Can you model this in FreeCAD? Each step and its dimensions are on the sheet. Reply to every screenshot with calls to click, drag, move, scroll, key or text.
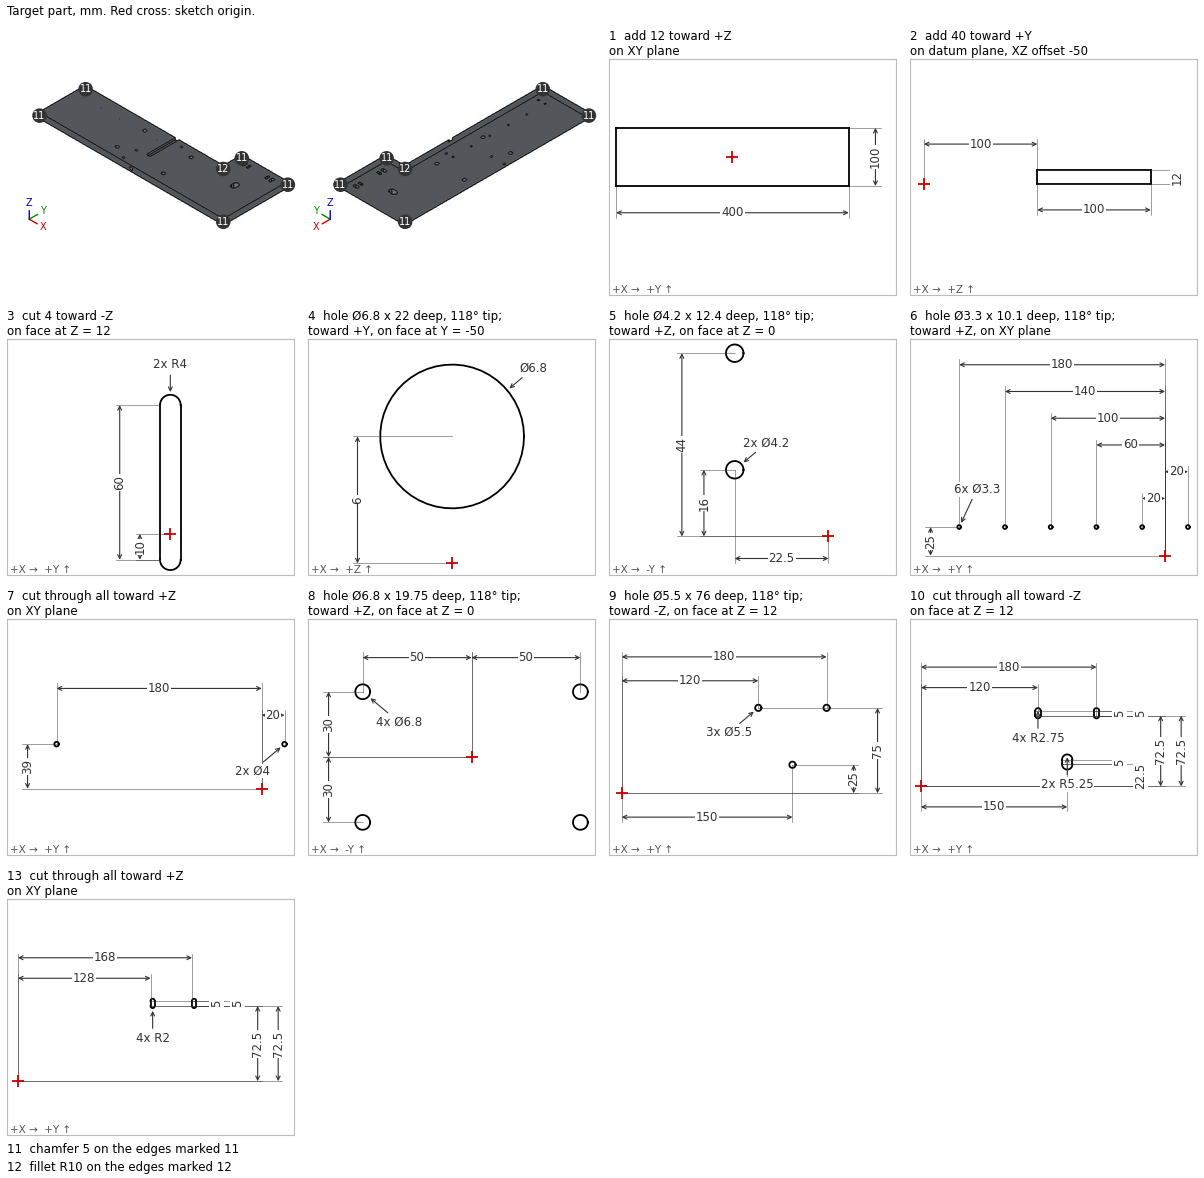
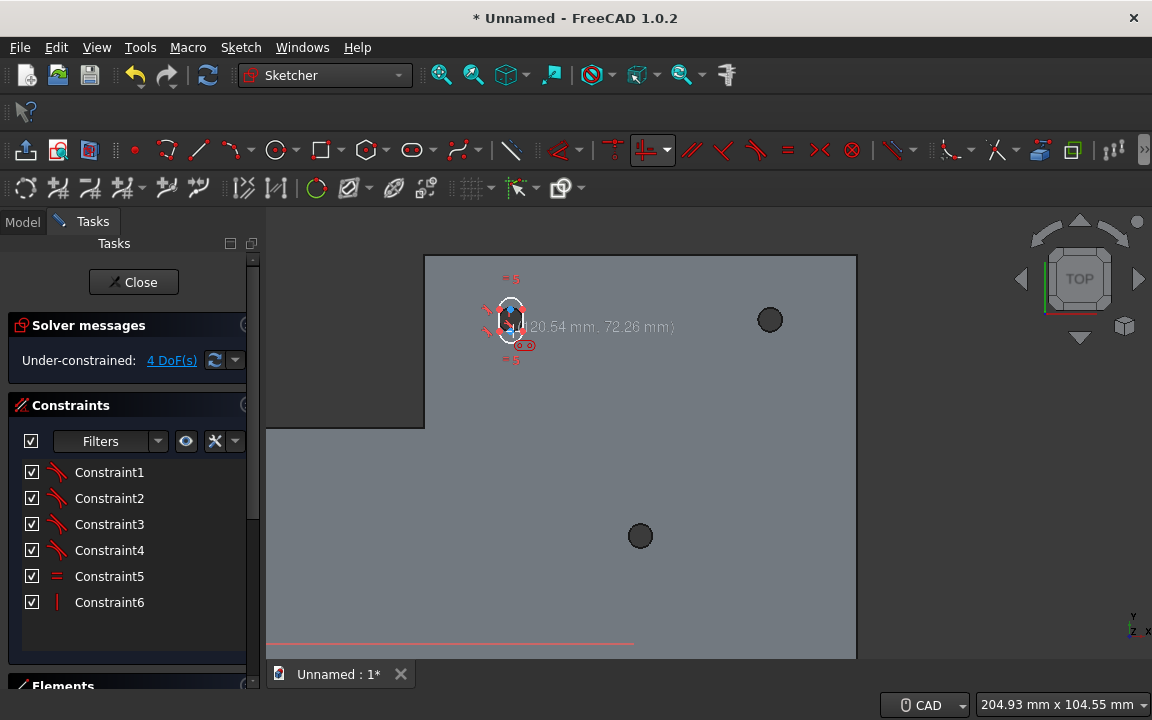
scroll(770, 331, up, 4)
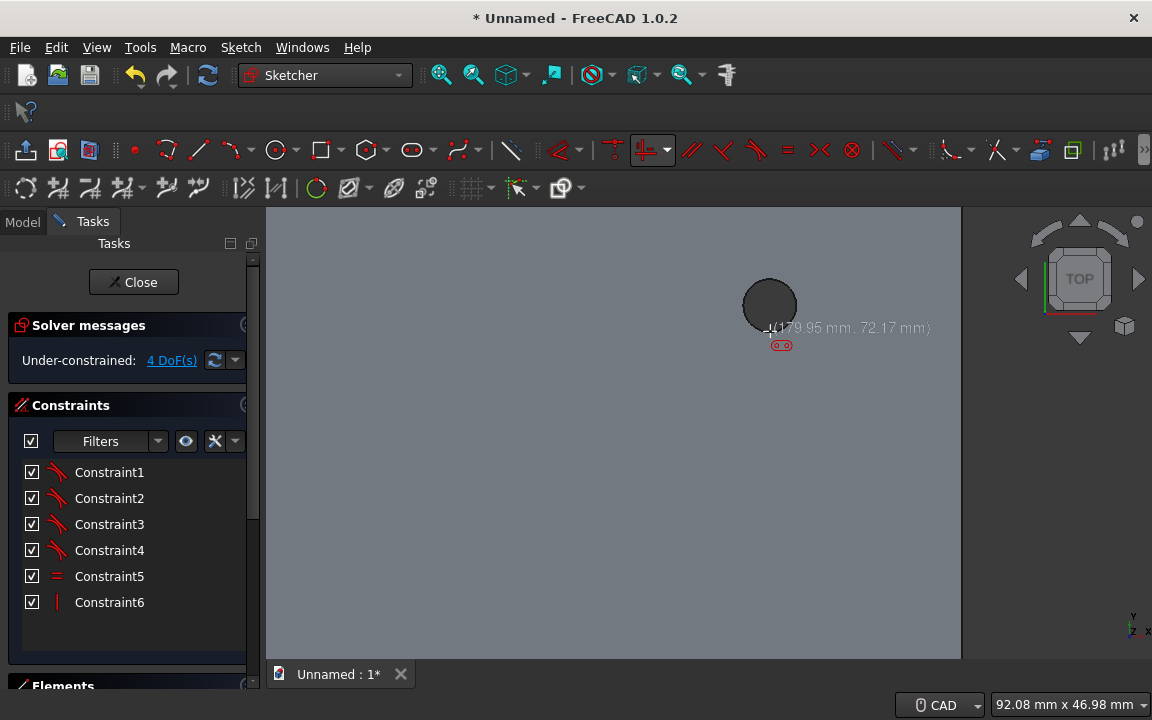
click(770, 330)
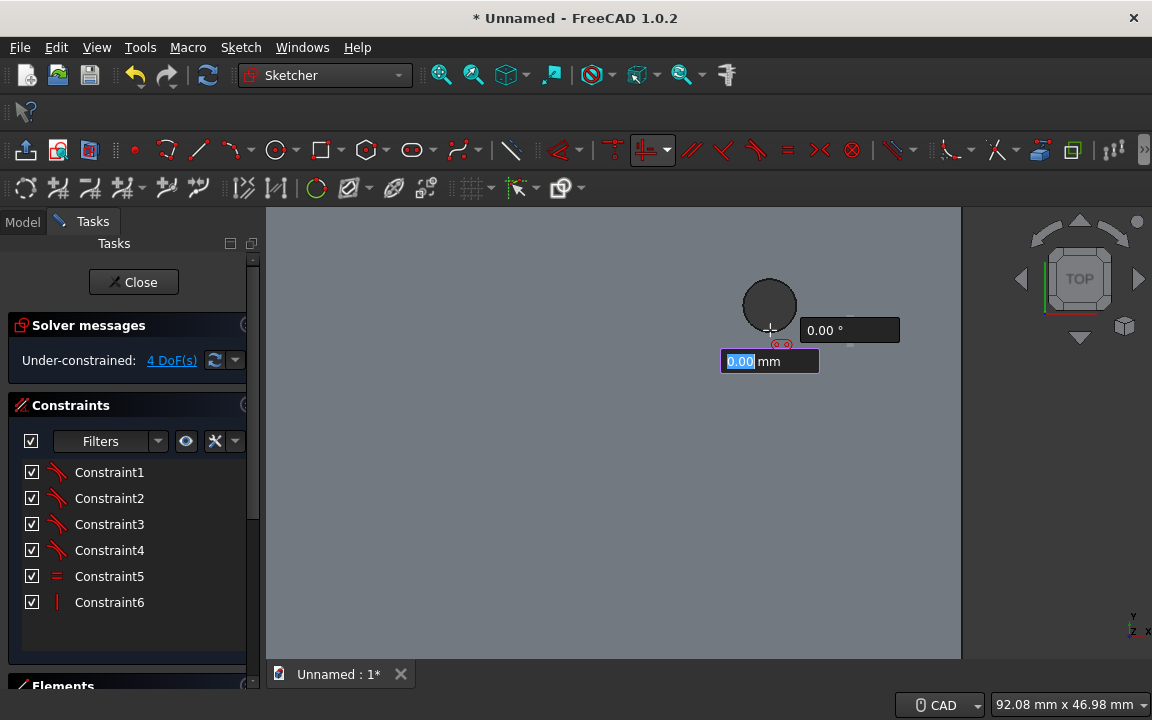
click(770, 282)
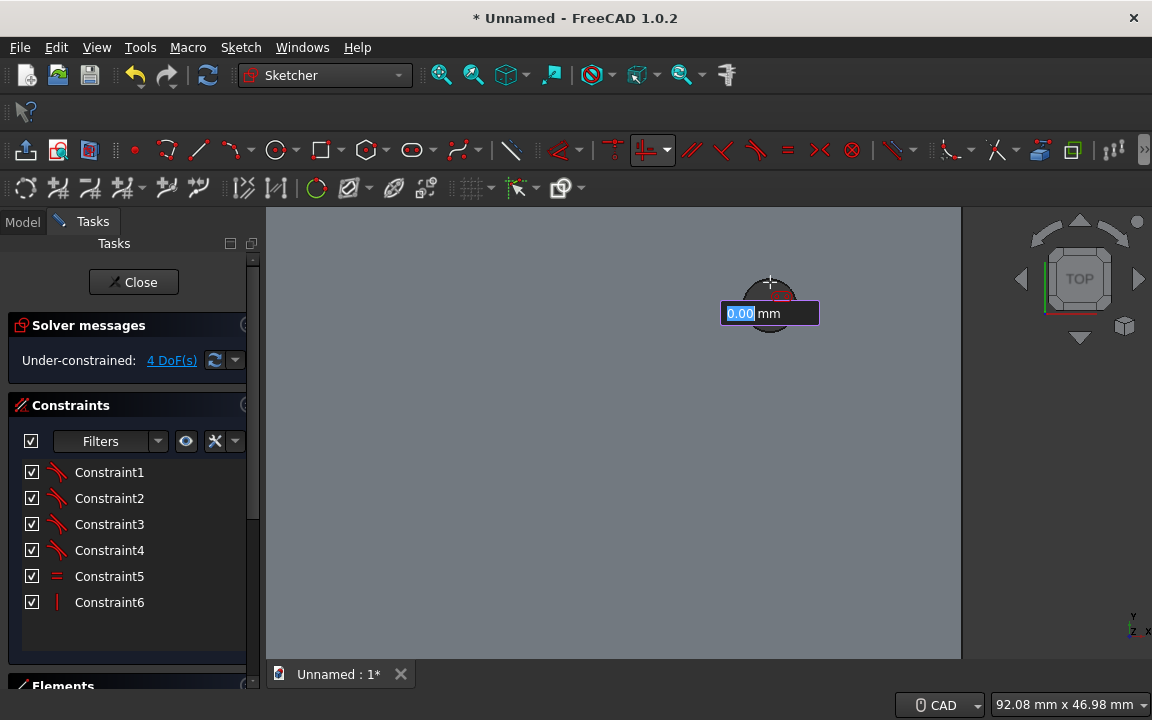
click(796, 306)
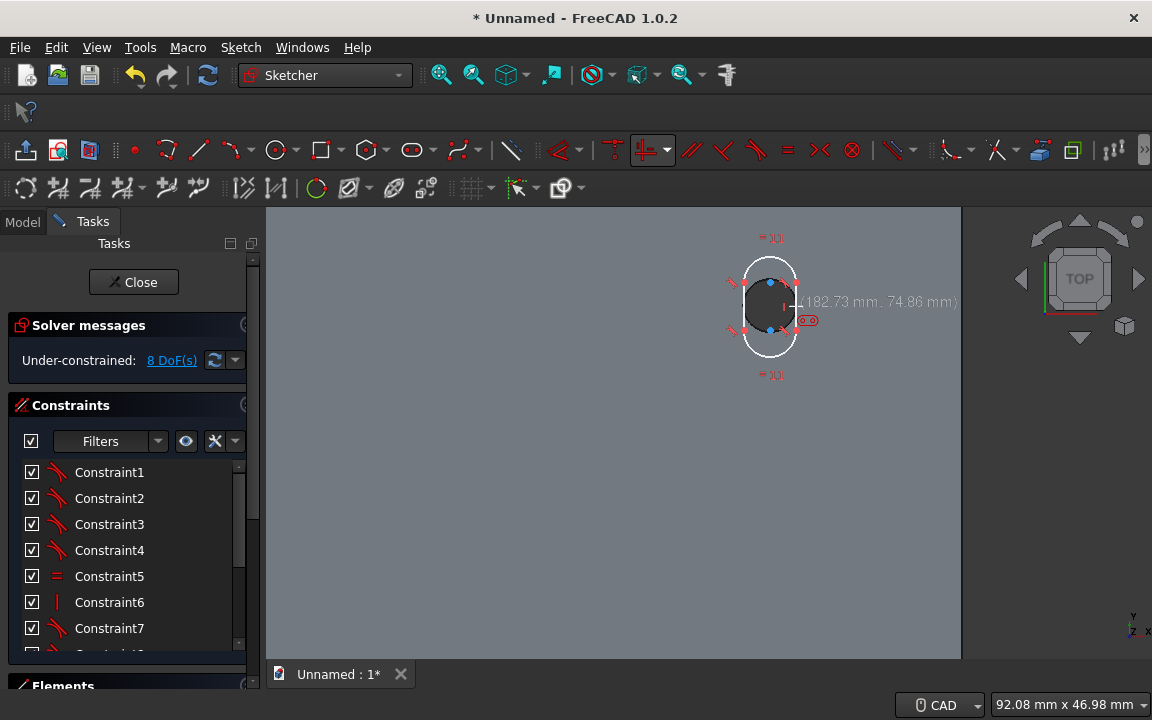
scroll(771, 331, down, 4)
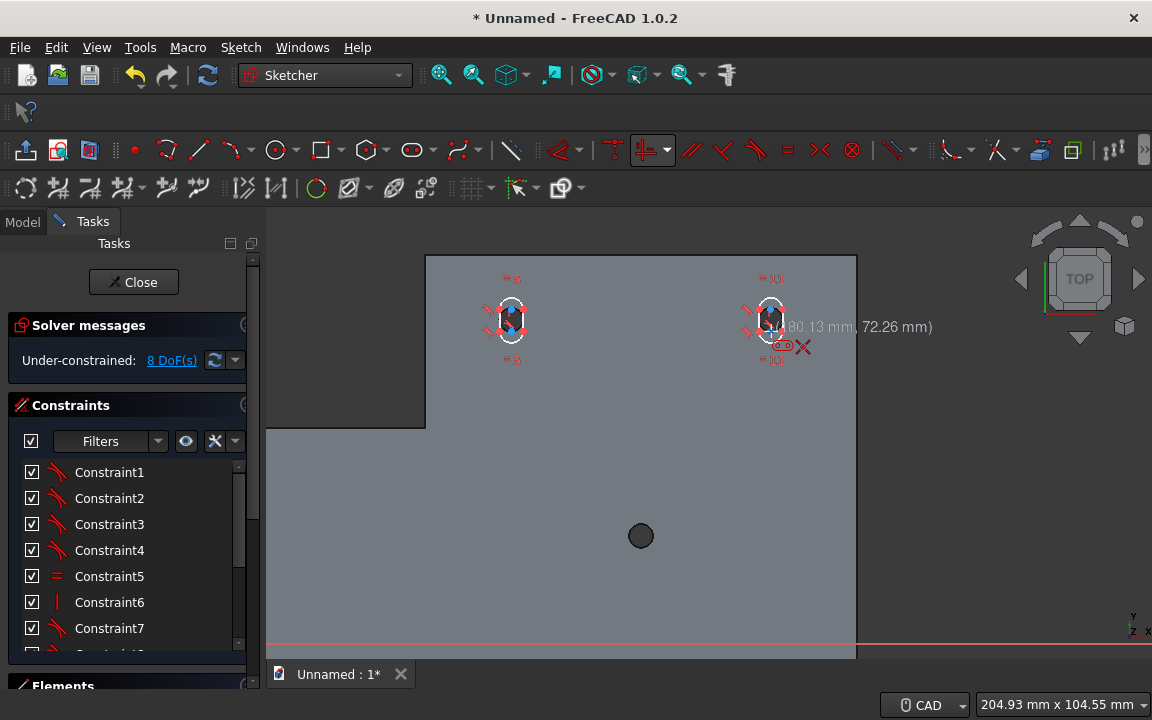
click(641, 547)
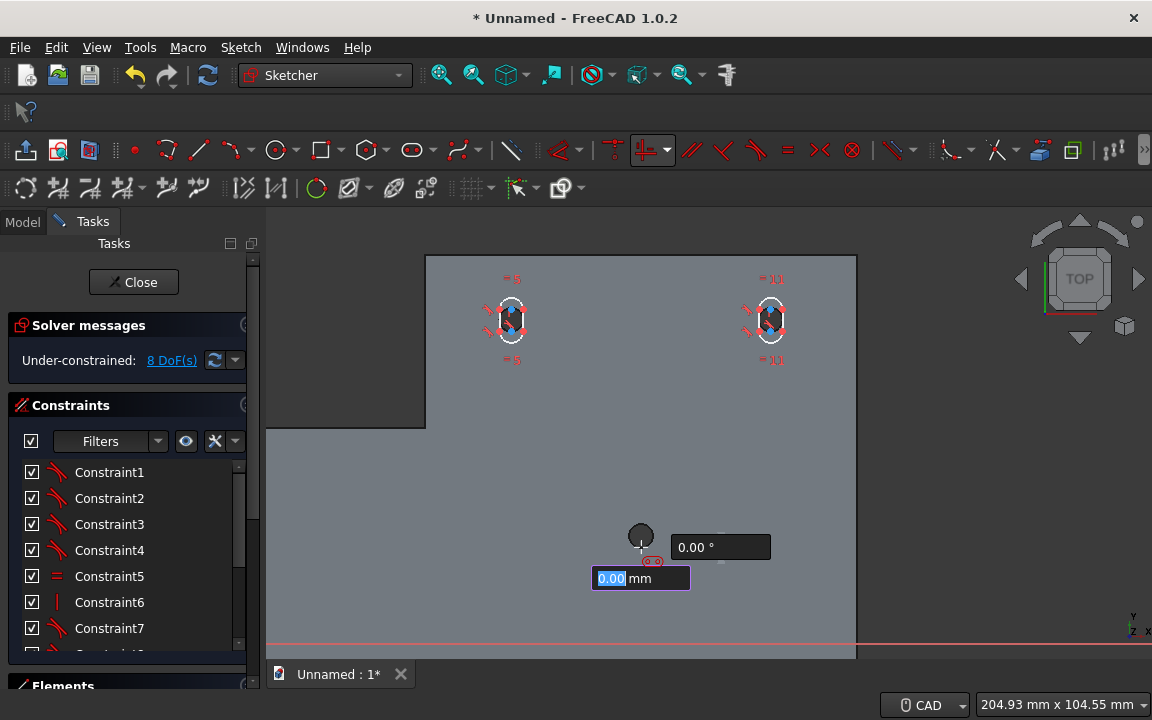
click(641, 525)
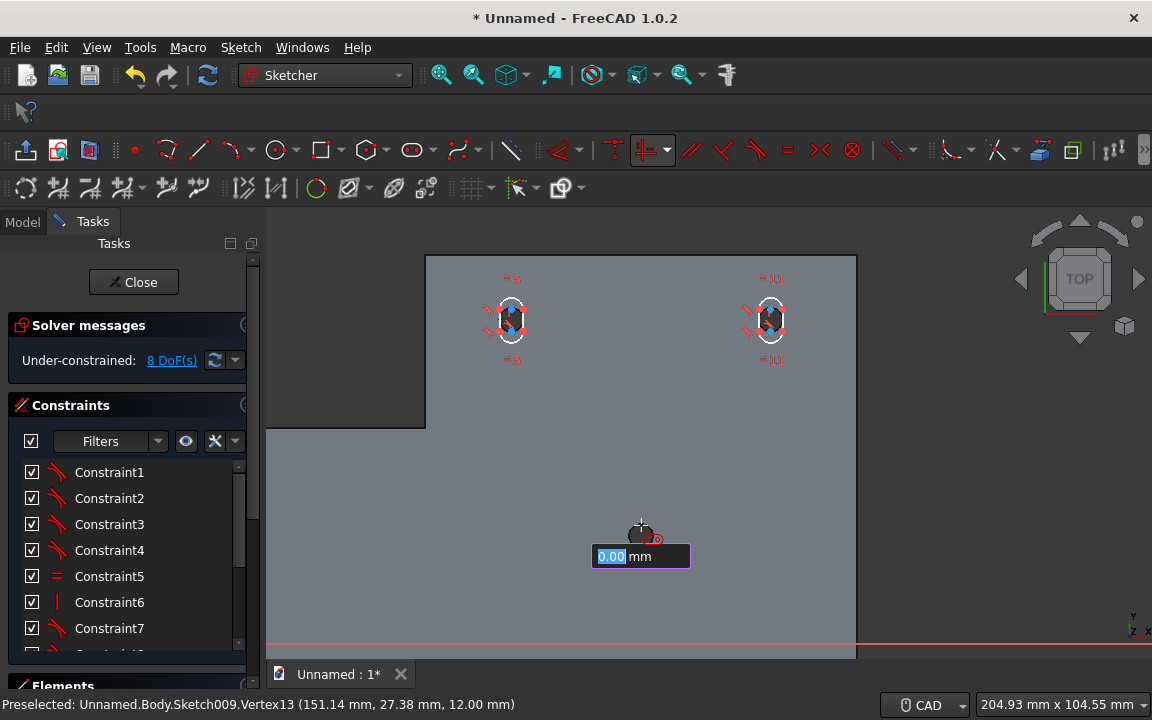
click(664, 536)
key(Escape)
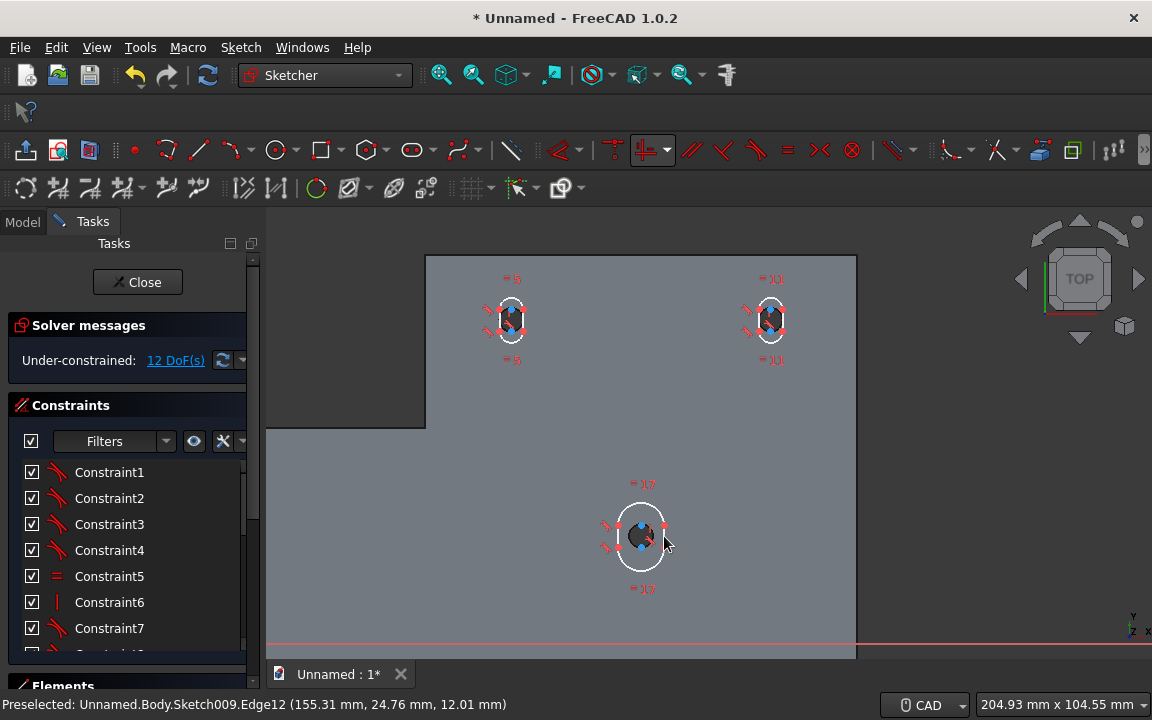
scroll(505, 341, up, 2)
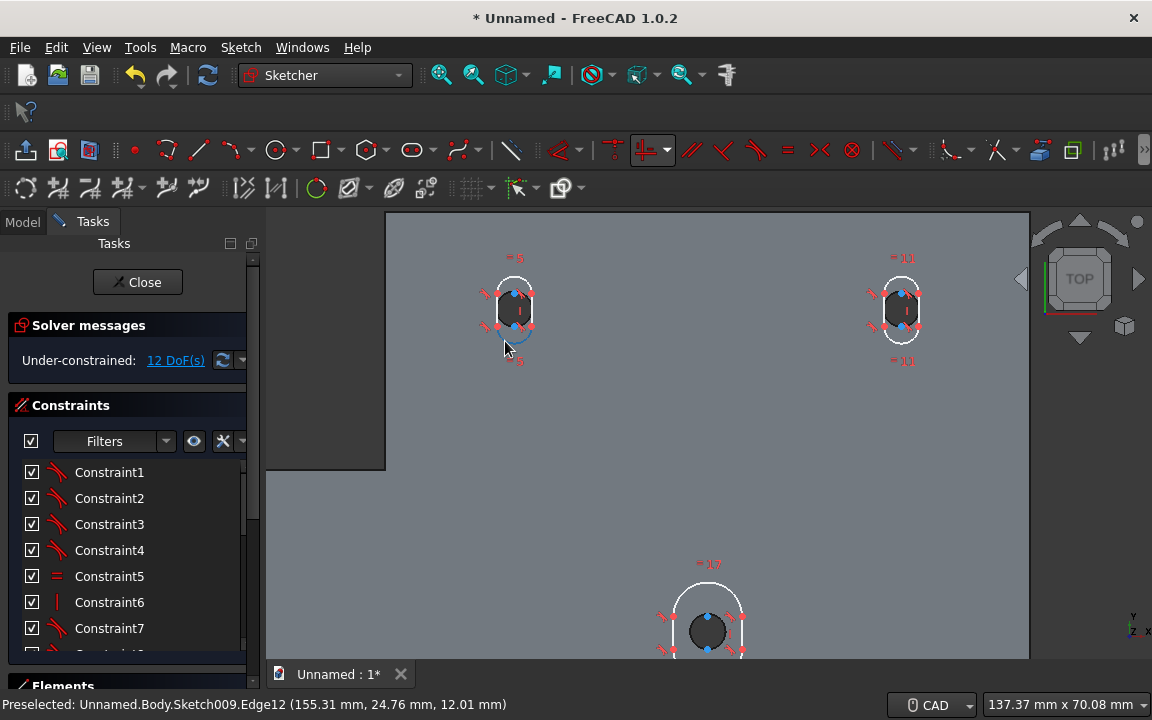
click(504, 340)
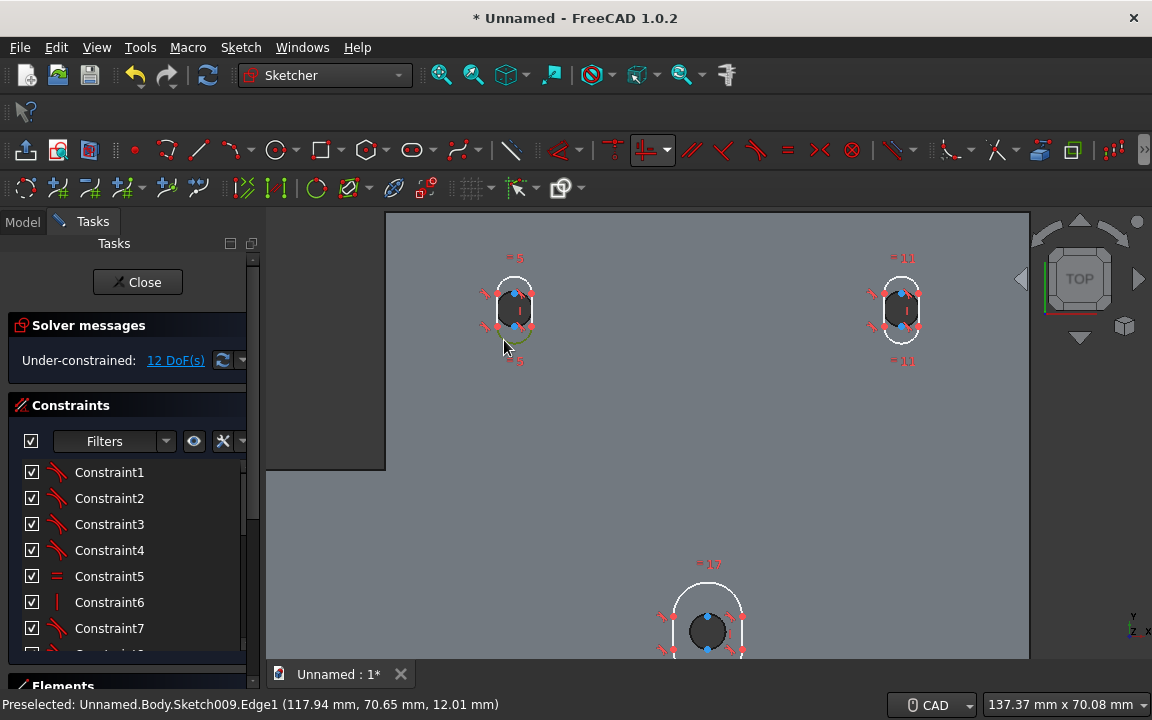
click(891, 340)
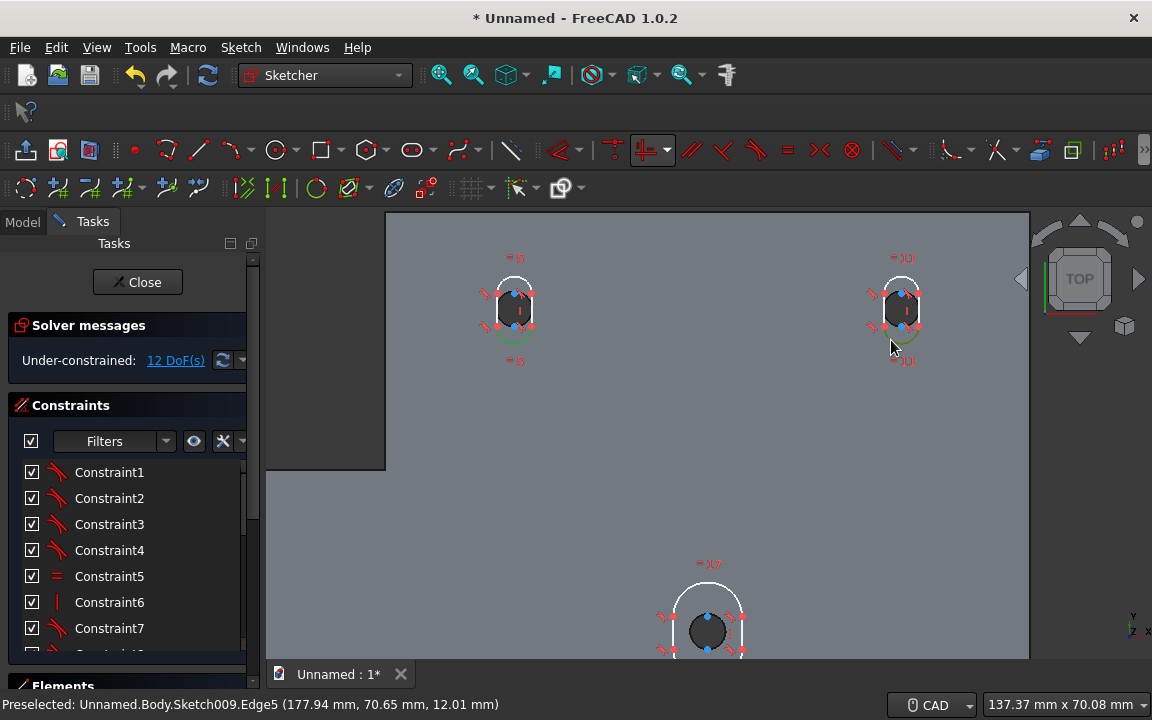
click(788, 150)